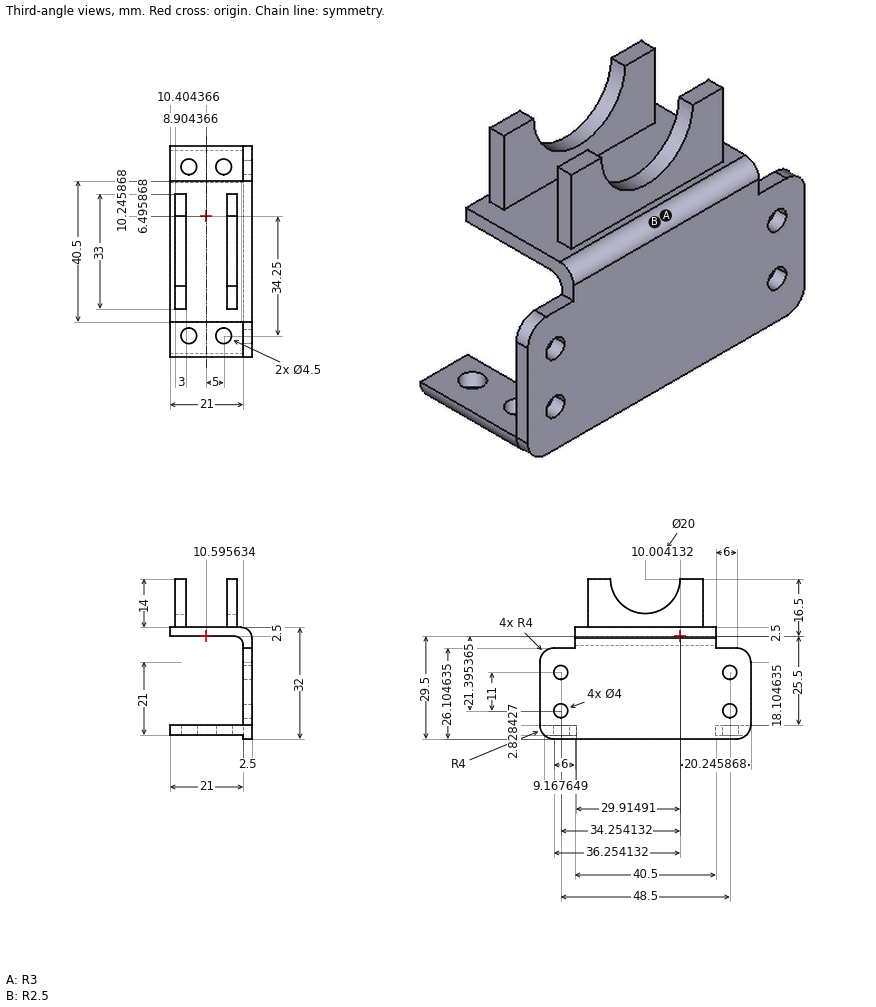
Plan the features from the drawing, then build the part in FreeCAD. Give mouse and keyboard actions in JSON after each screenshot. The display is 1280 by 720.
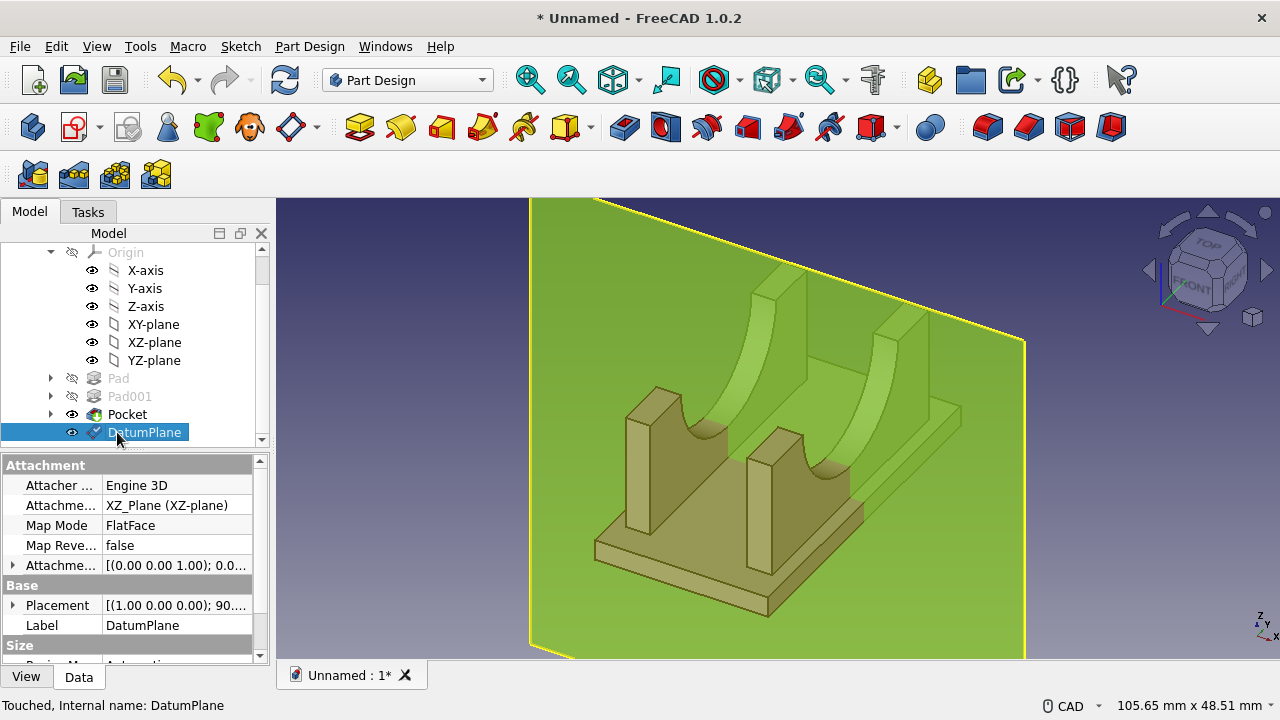
{"action": "left_click", "coordinate": [74, 128]}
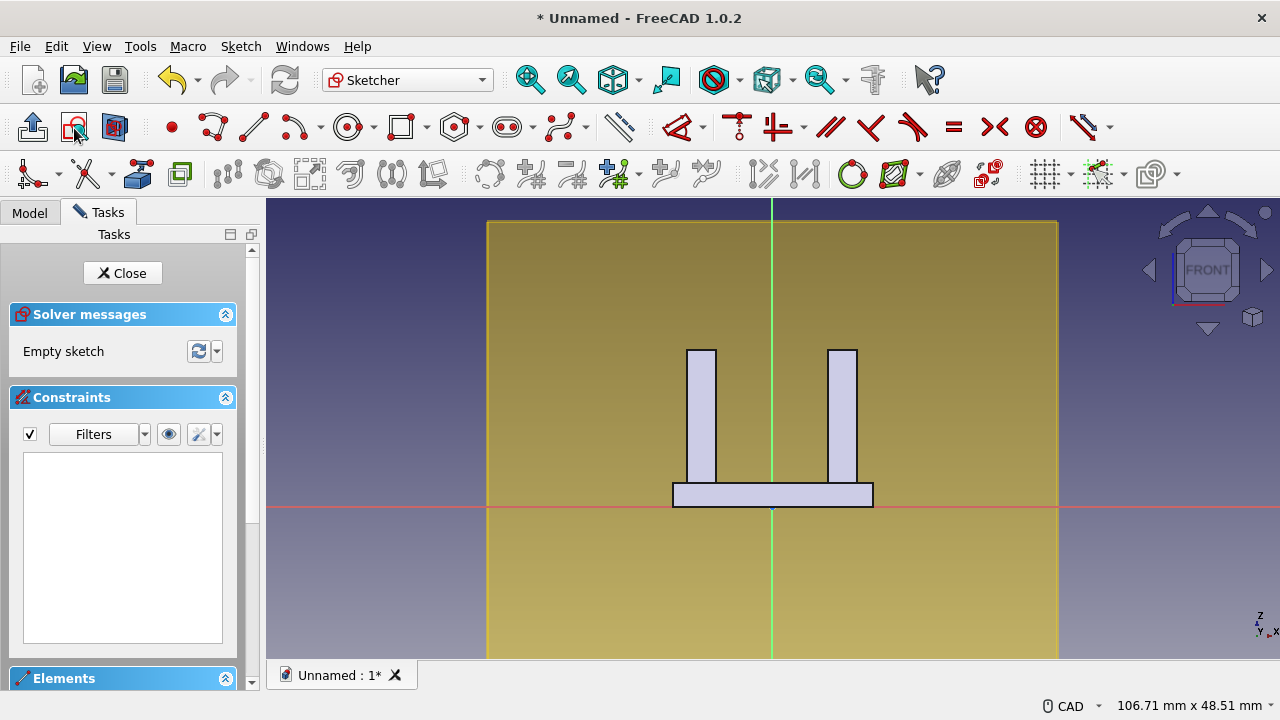
{"action": "left_click", "coordinate": [115, 128]}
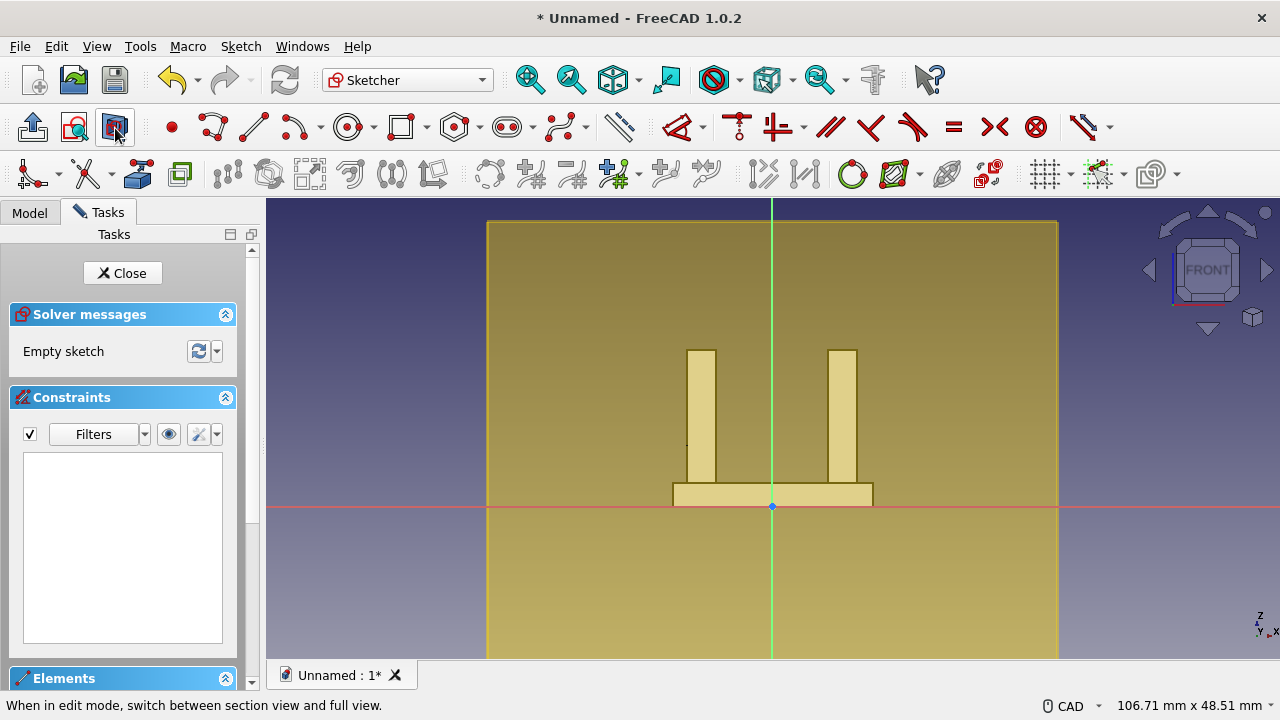
{"action": "scroll", "coordinate": [441, 226], "scroll_direction": "down", "scroll_amount": 2}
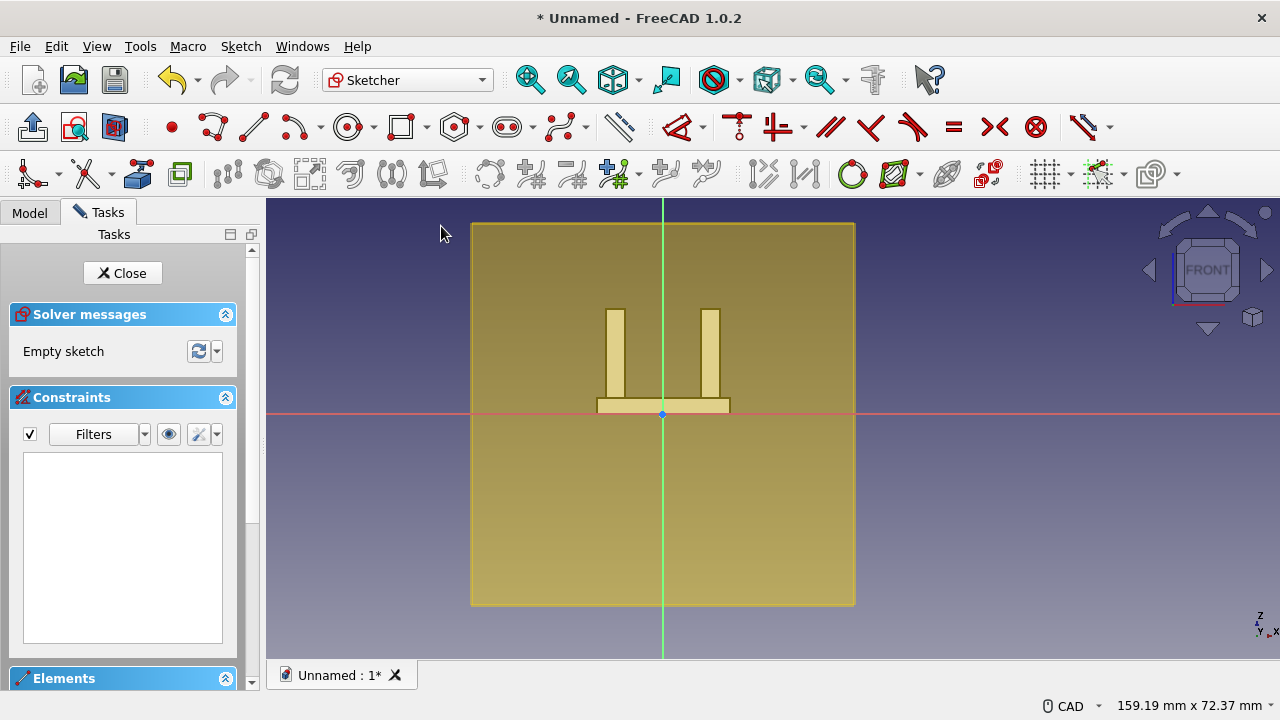
{"action": "scroll", "coordinate": [705, 631], "scroll_direction": "up", "scroll_amount": 2}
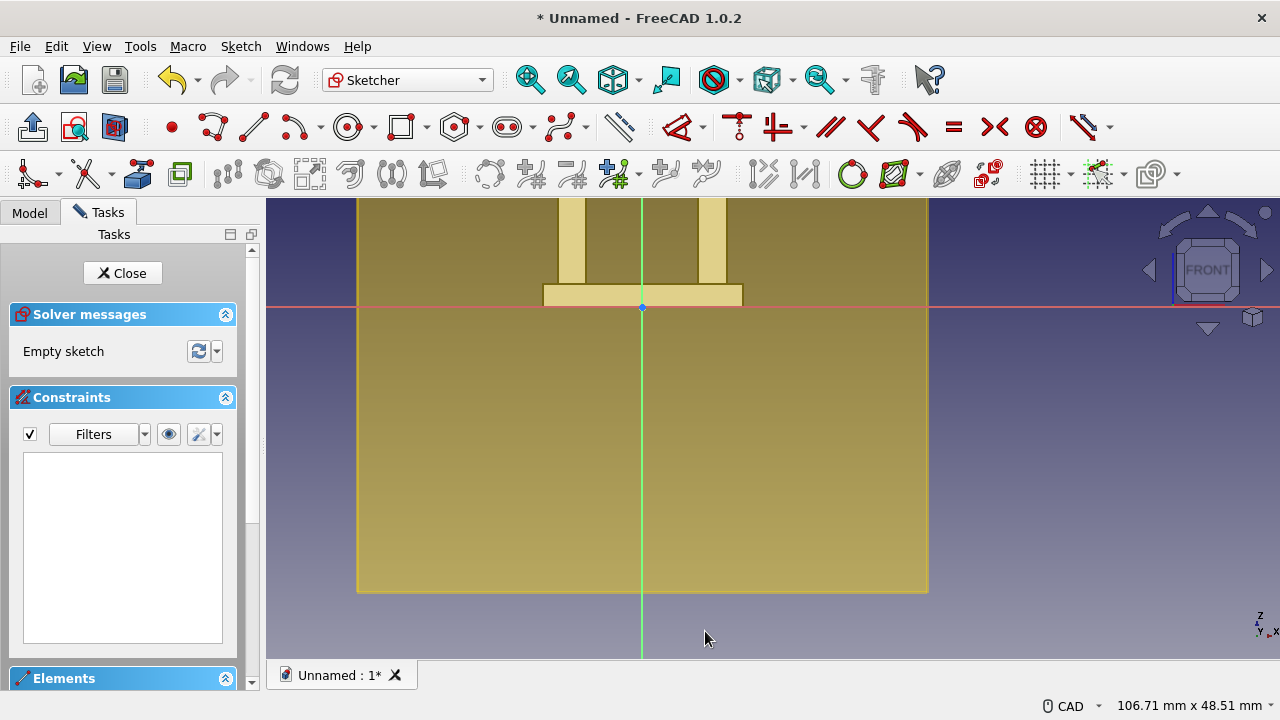
{"action": "left_click", "coordinate": [400, 128]}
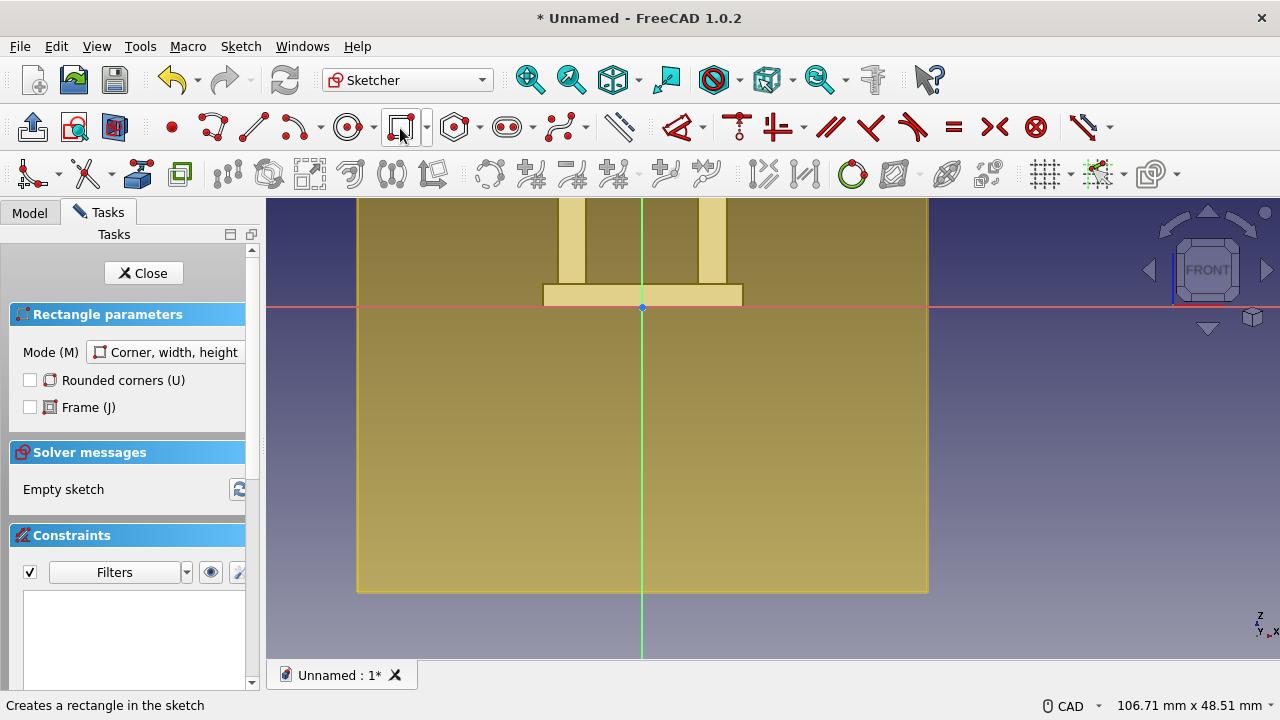
{"action": "left_click", "coordinate": [743, 284]}
{"action": "left_click", "coordinate": [767, 588]}
{"action": "key", "text": "Escape"}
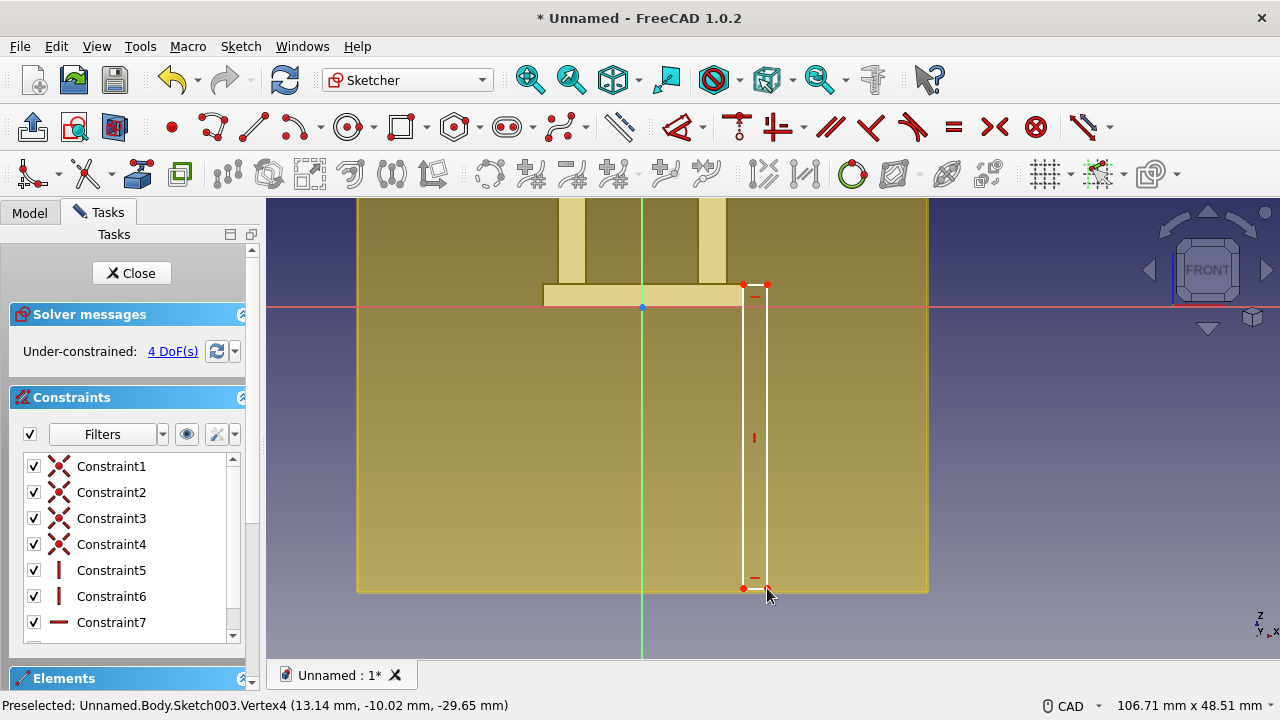
{"action": "left_click", "coordinate": [676, 128]}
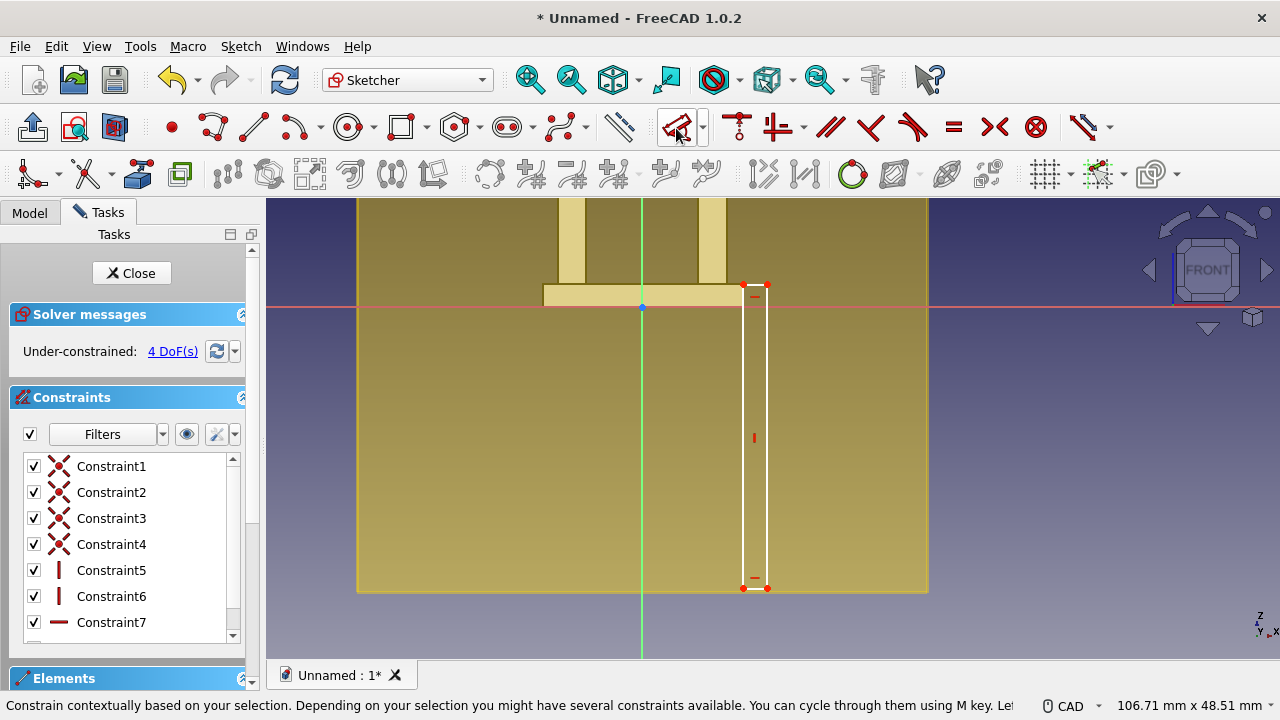
{"action": "left_click", "coordinate": [743, 376]}
{"action": "left_click", "coordinate": [709, 437]}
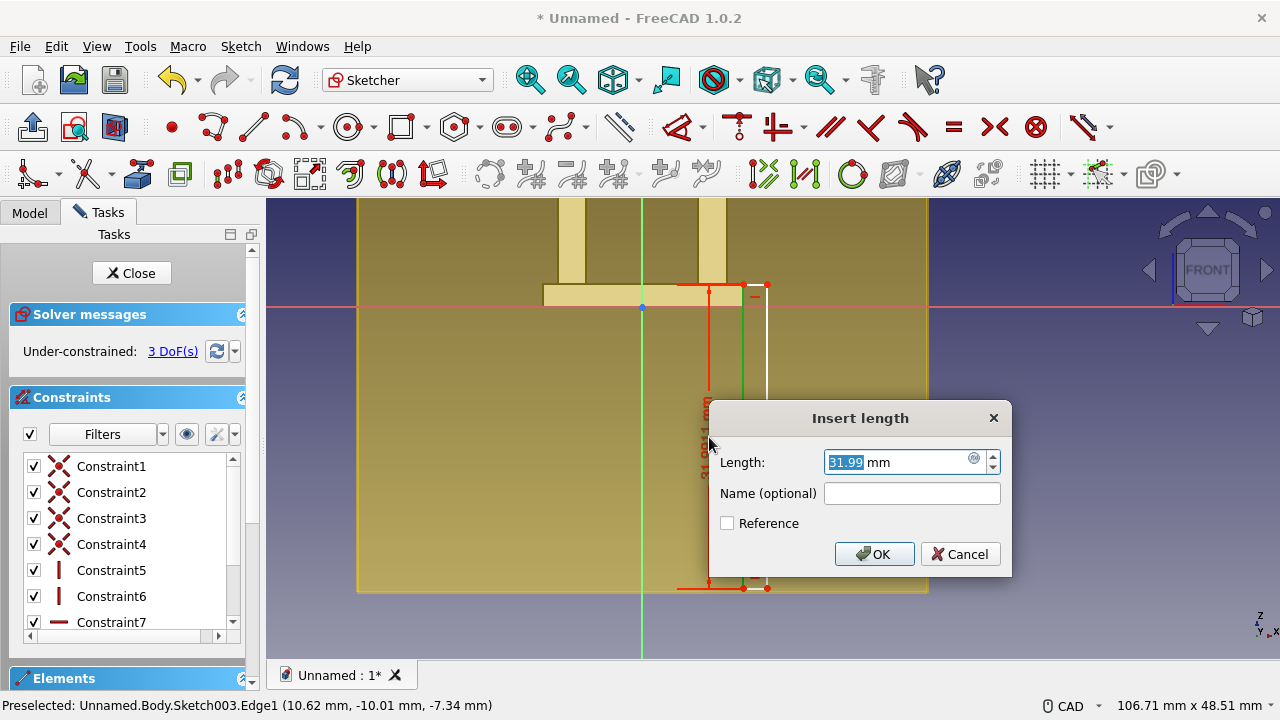
{"action": "type", "text": "32"}
{"action": "key", "text": "Return"}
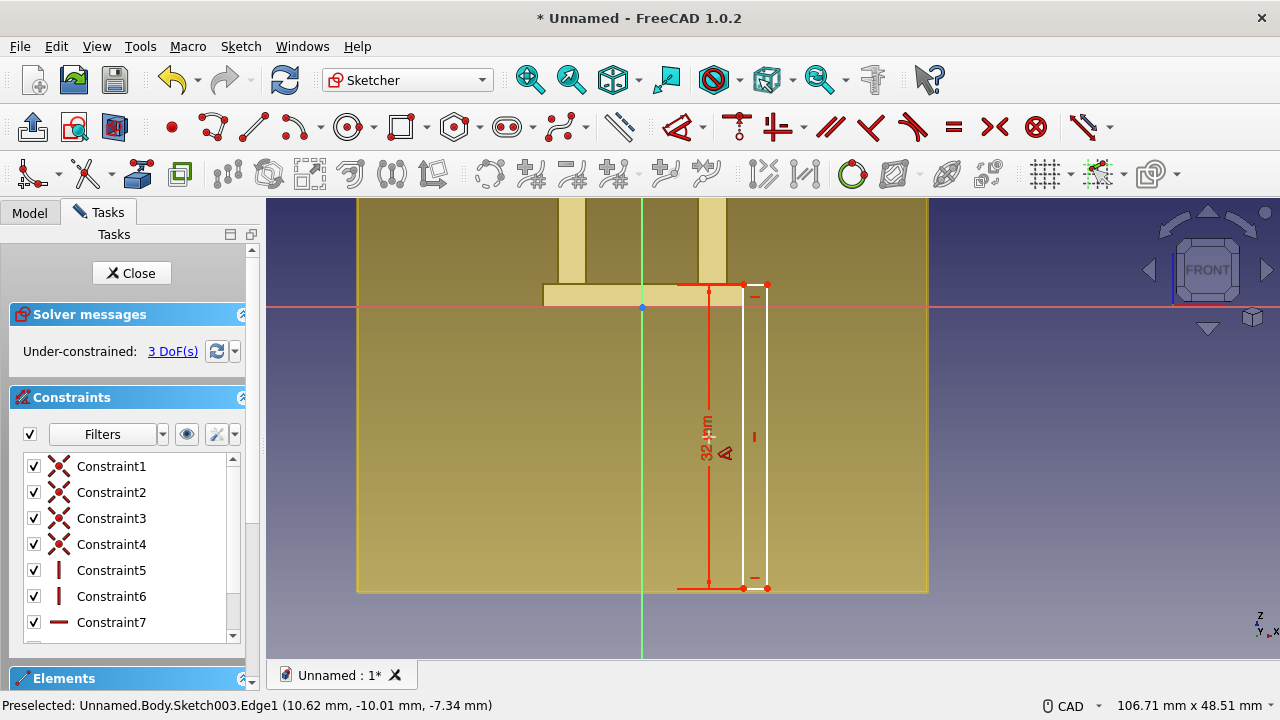
{"action": "scroll", "coordinate": [753, 589], "scroll_direction": "up", "scroll_amount": 3}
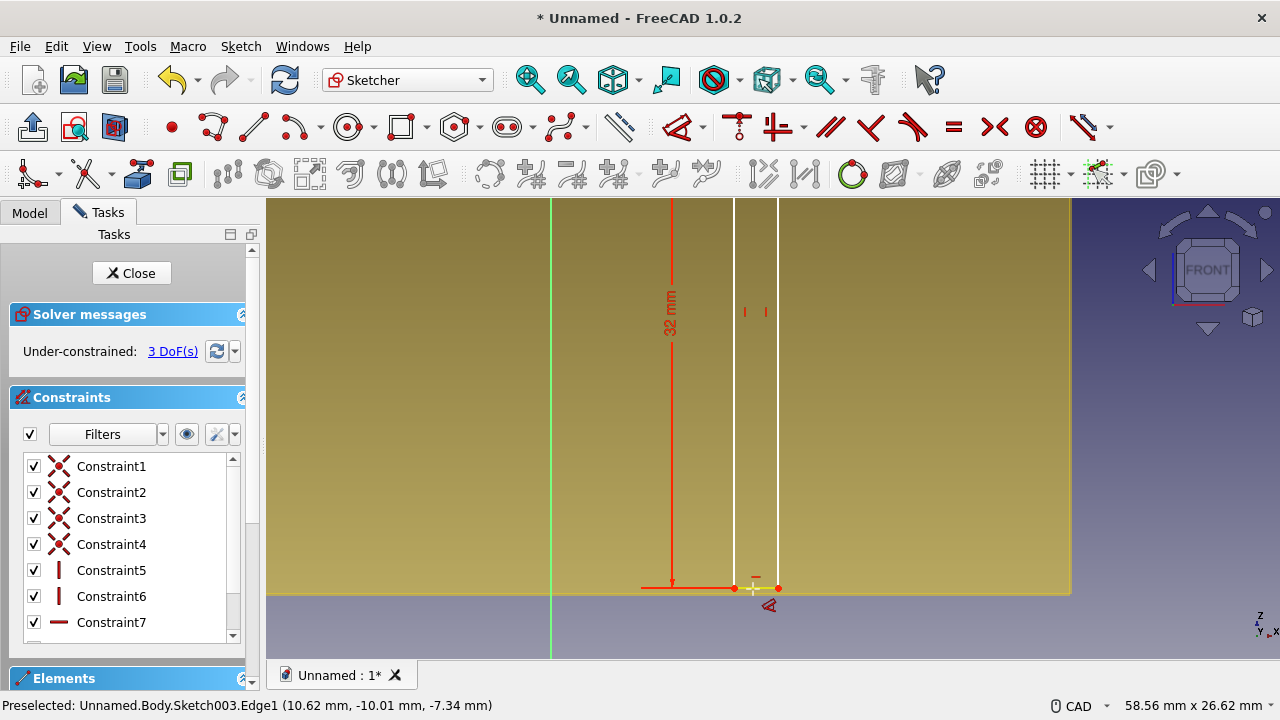
{"action": "left_click", "coordinate": [752, 588]}
{"action": "left_click", "coordinate": [756, 622]}